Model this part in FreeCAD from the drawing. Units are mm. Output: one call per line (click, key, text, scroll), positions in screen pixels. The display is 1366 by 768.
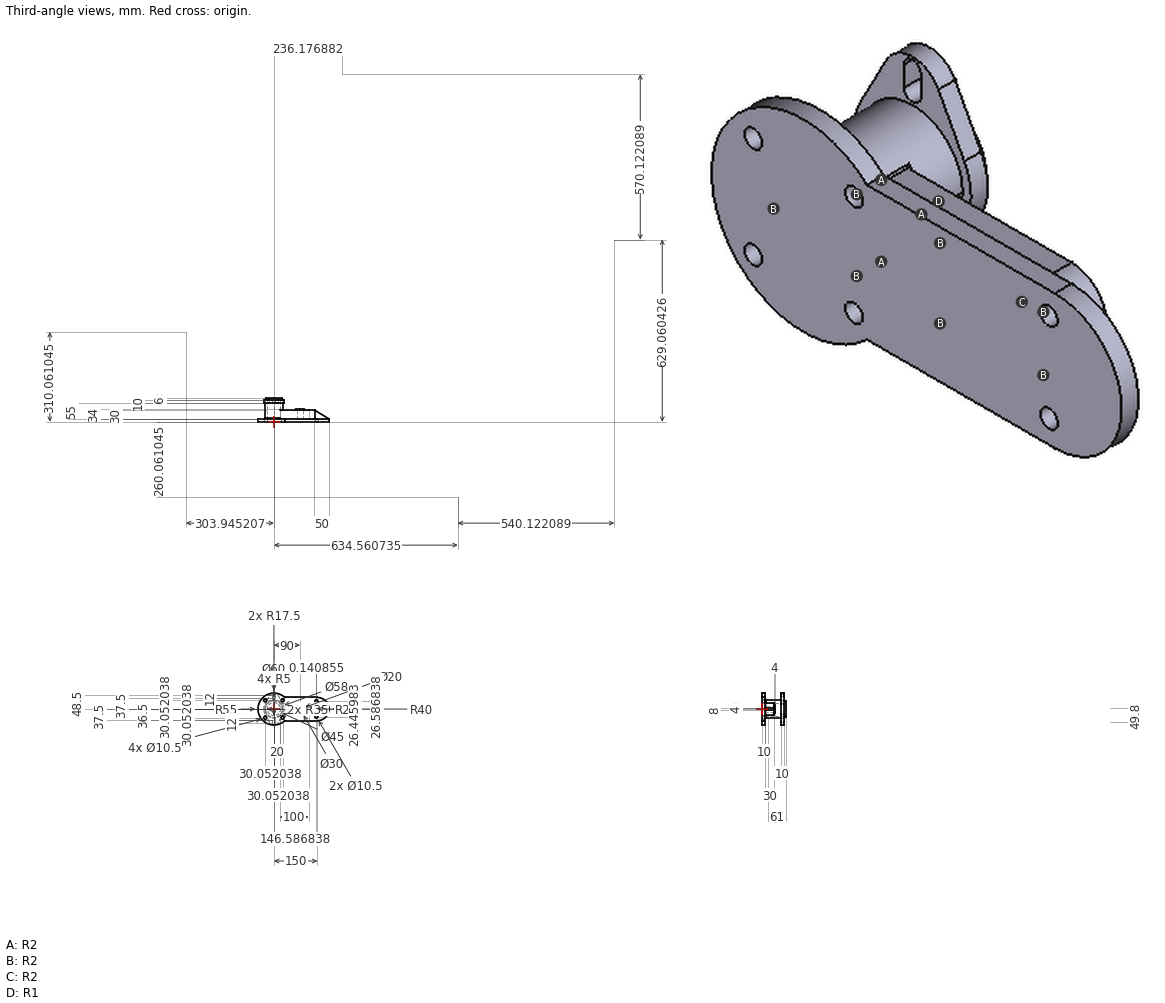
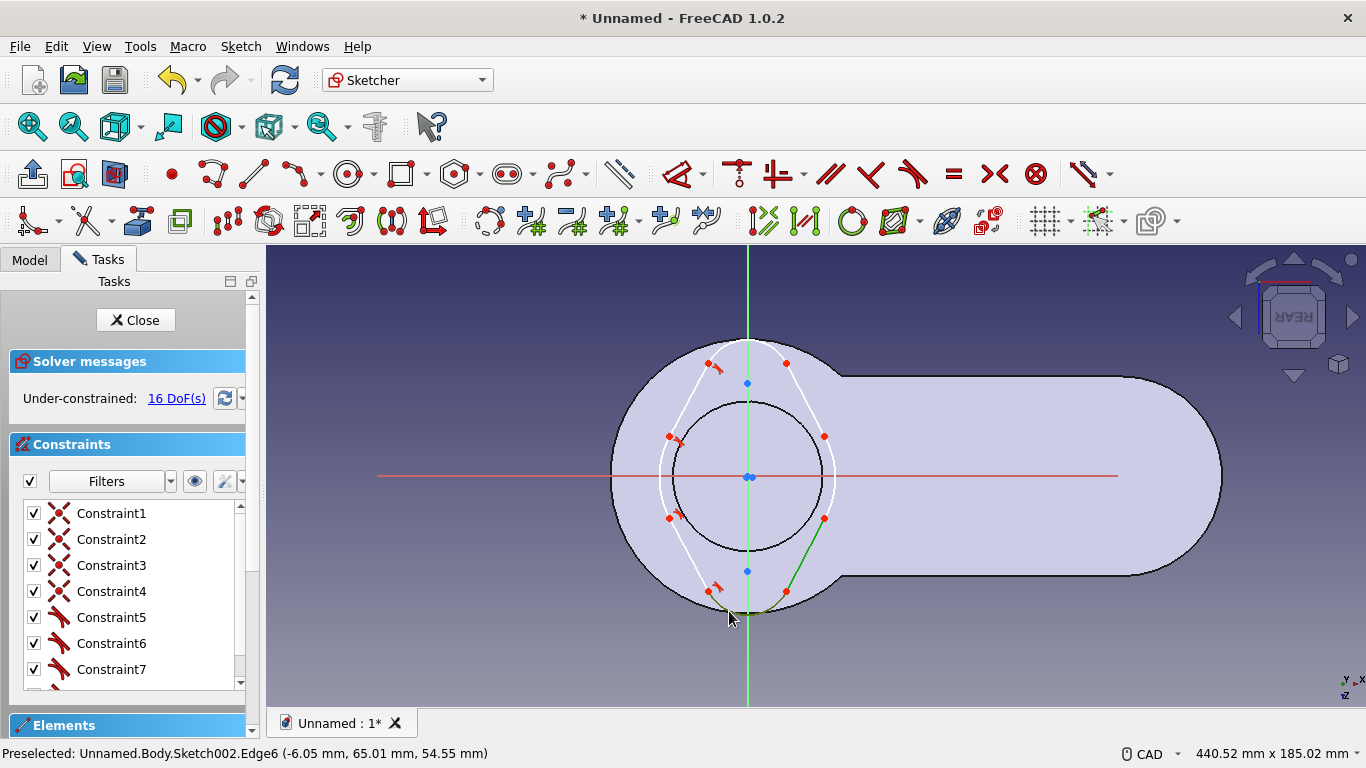
key(t)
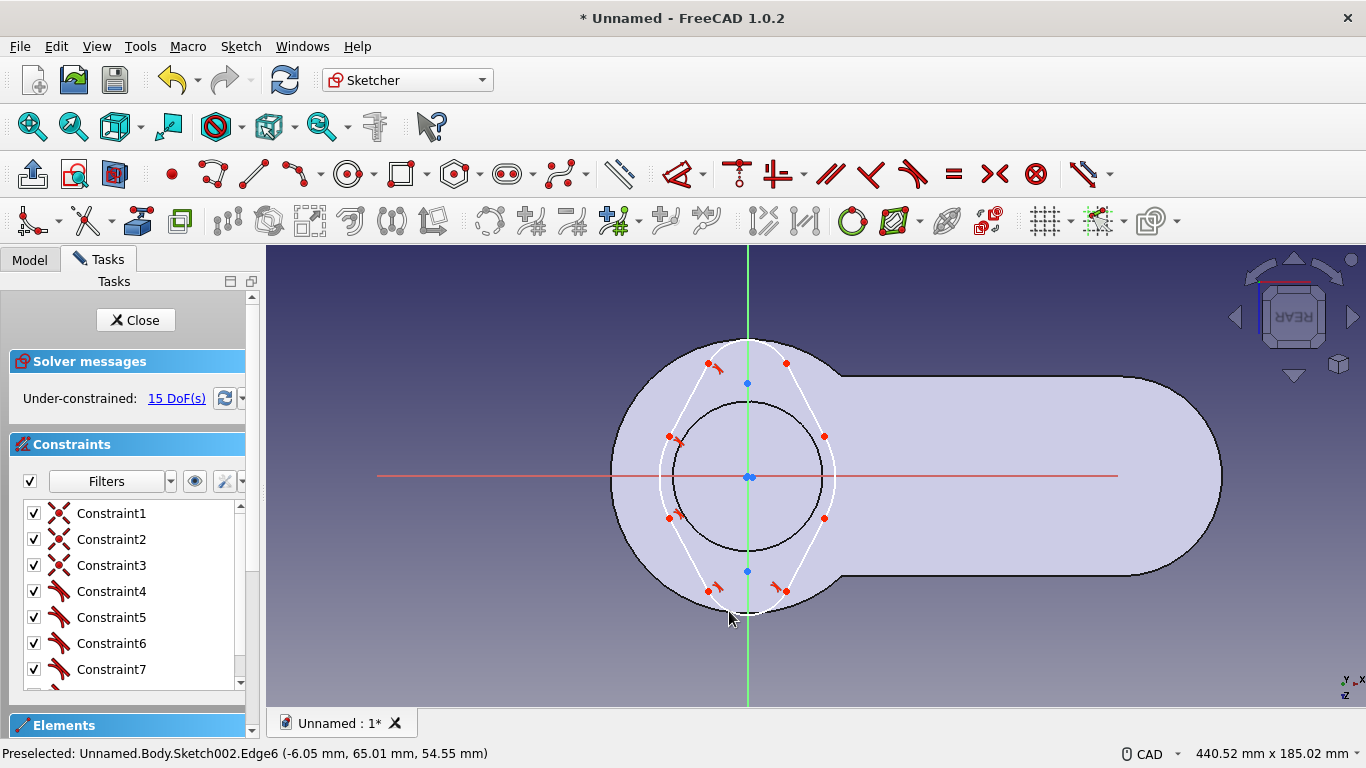
click(798, 570)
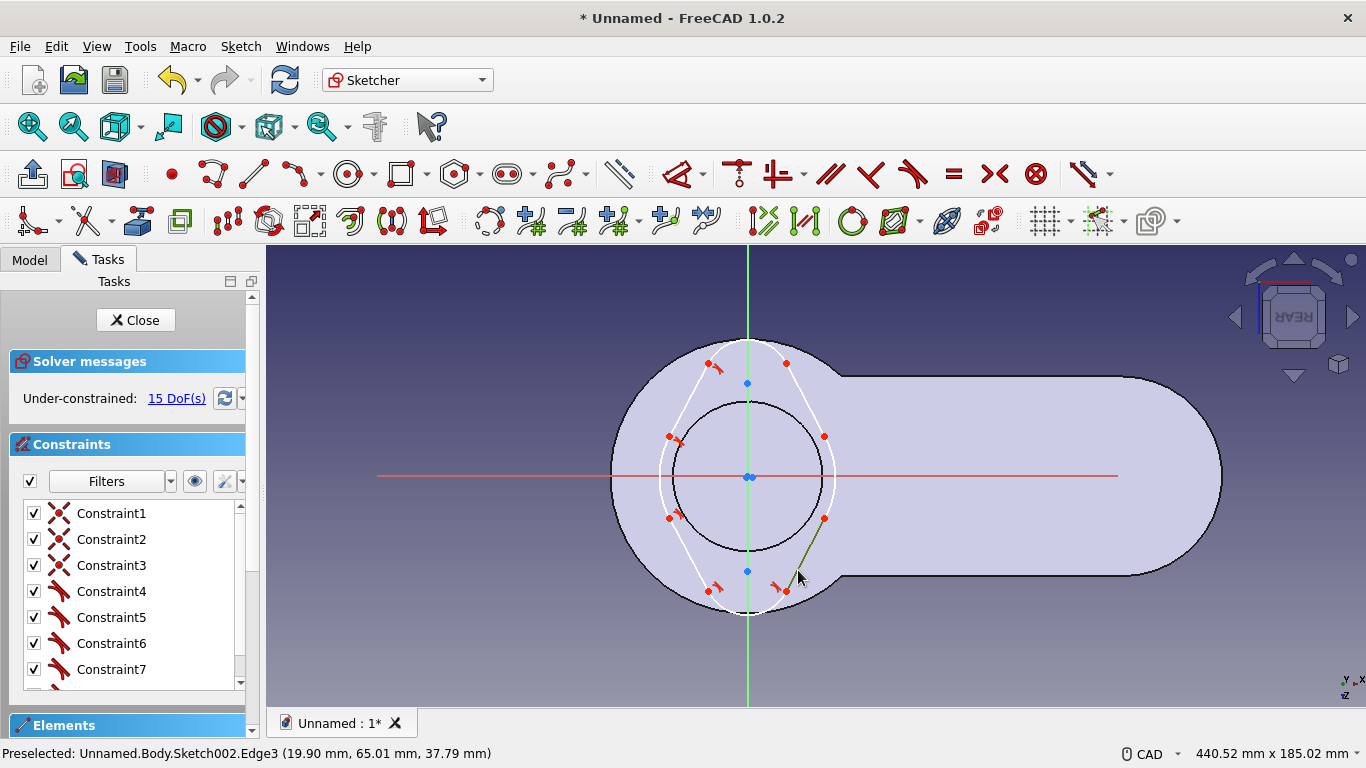
click(834, 495)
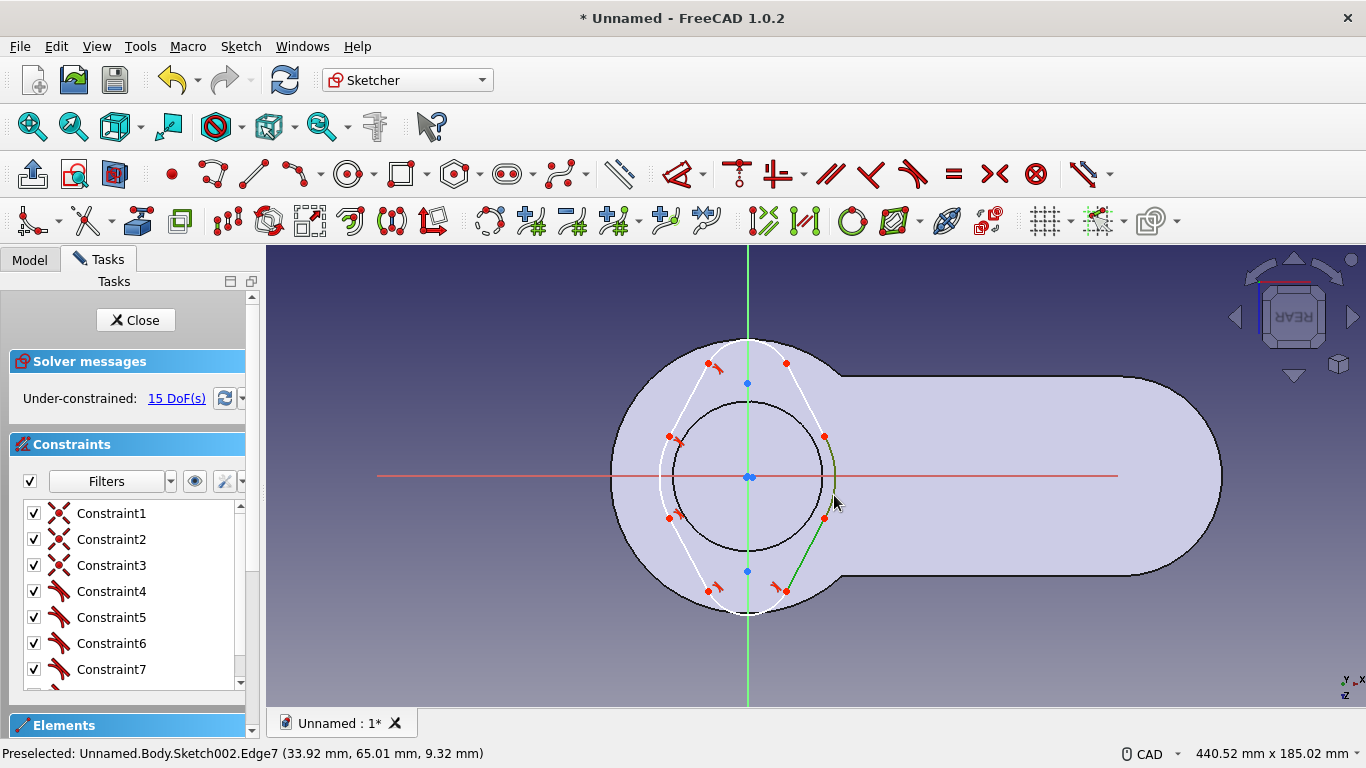
key(t)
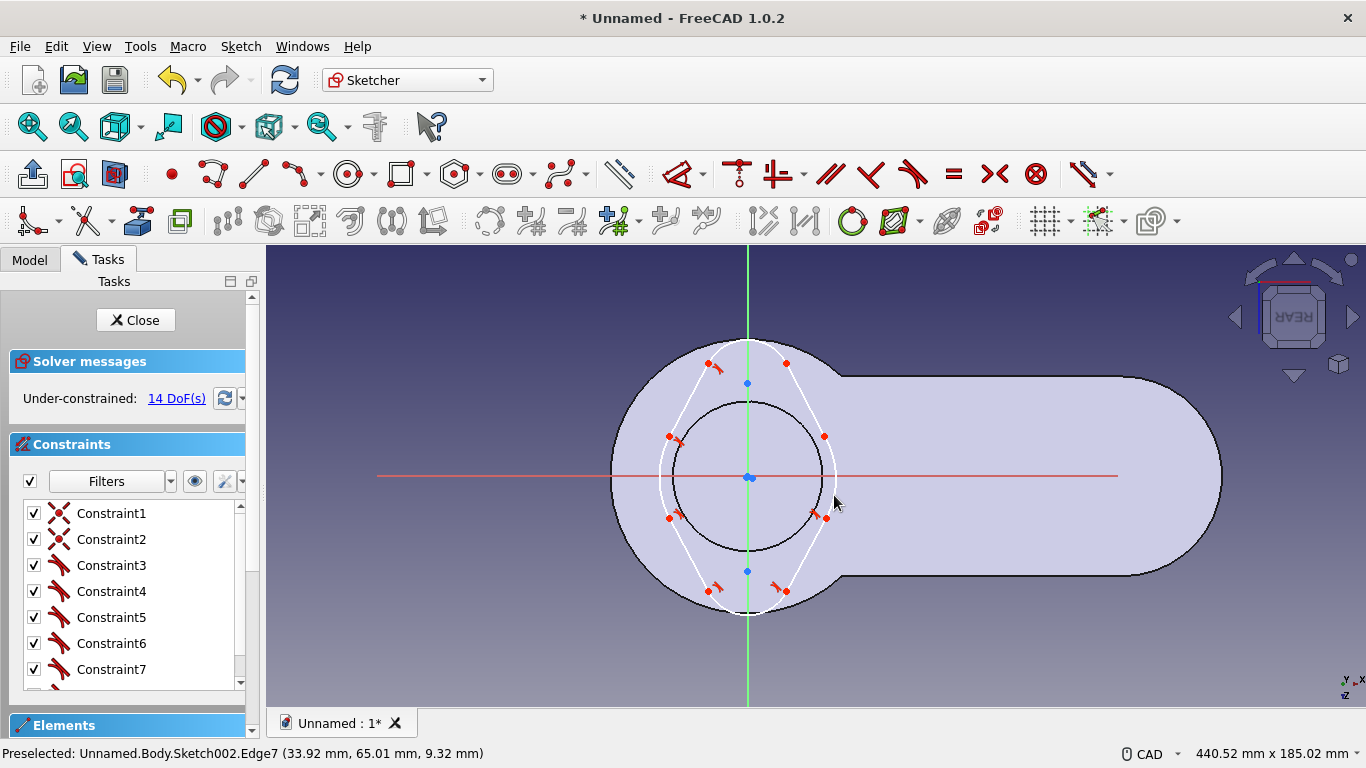
click(813, 415)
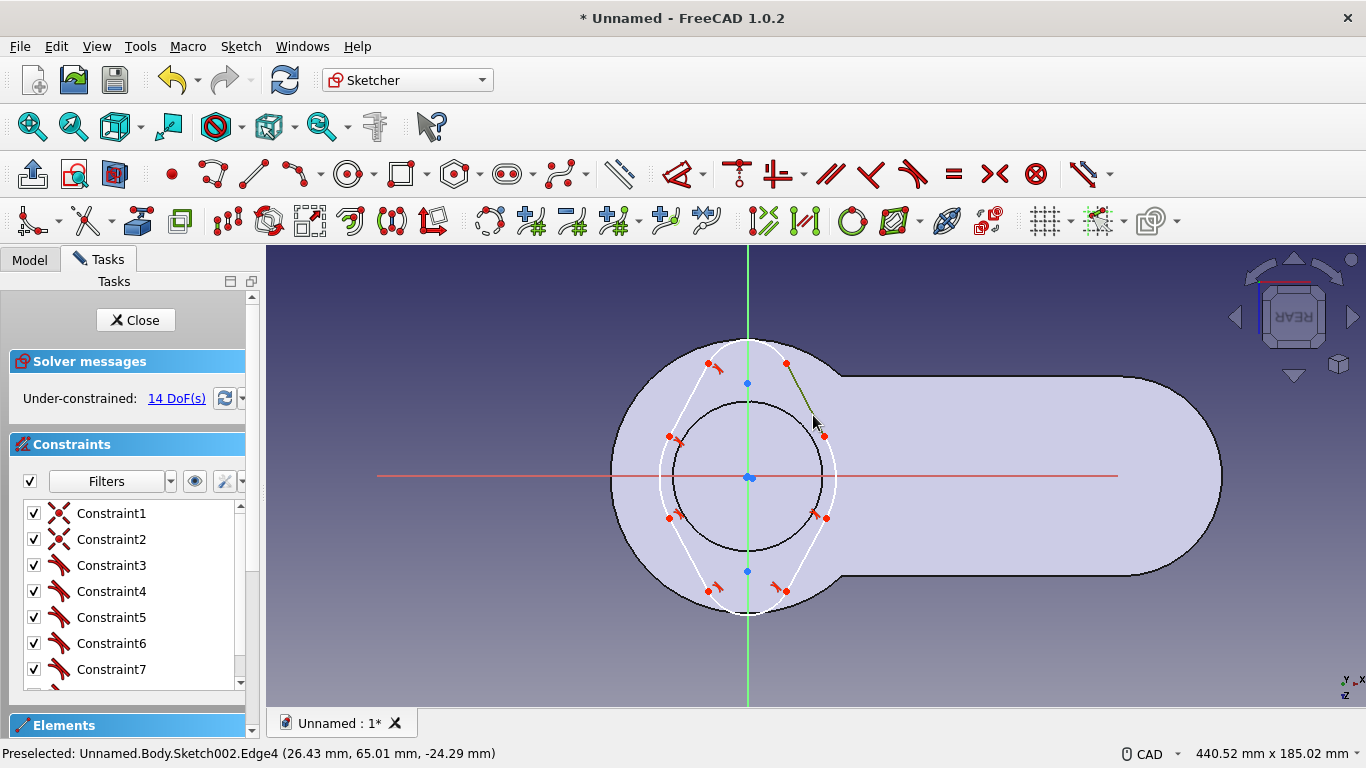
click(835, 494)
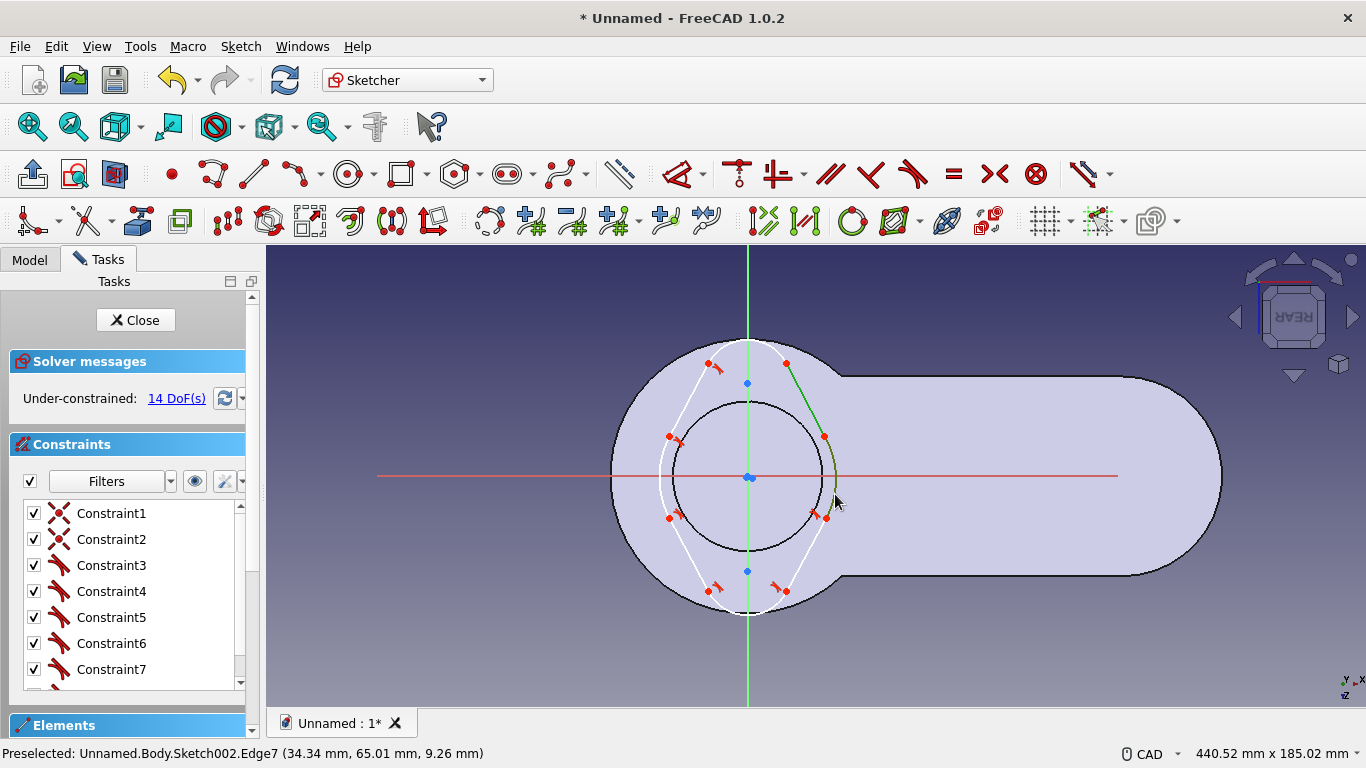
key(t)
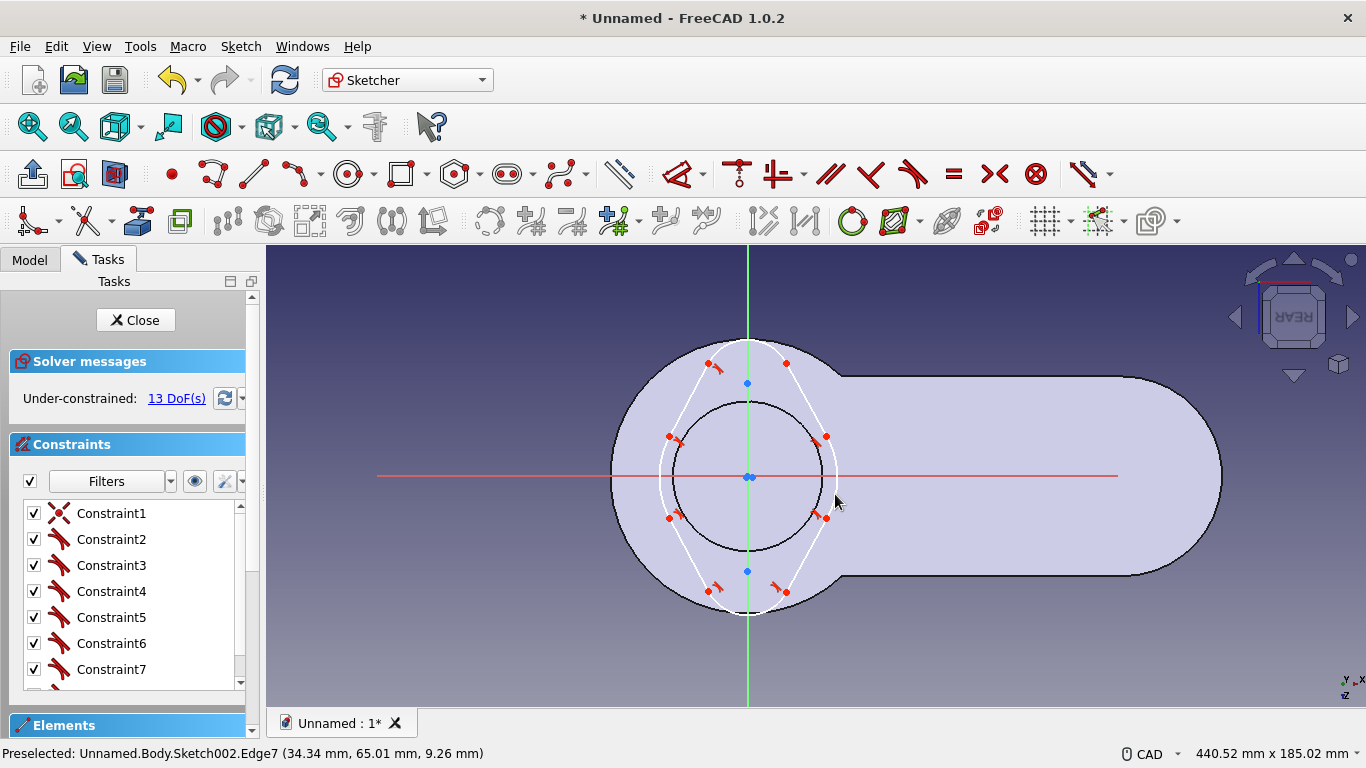
click(815, 415)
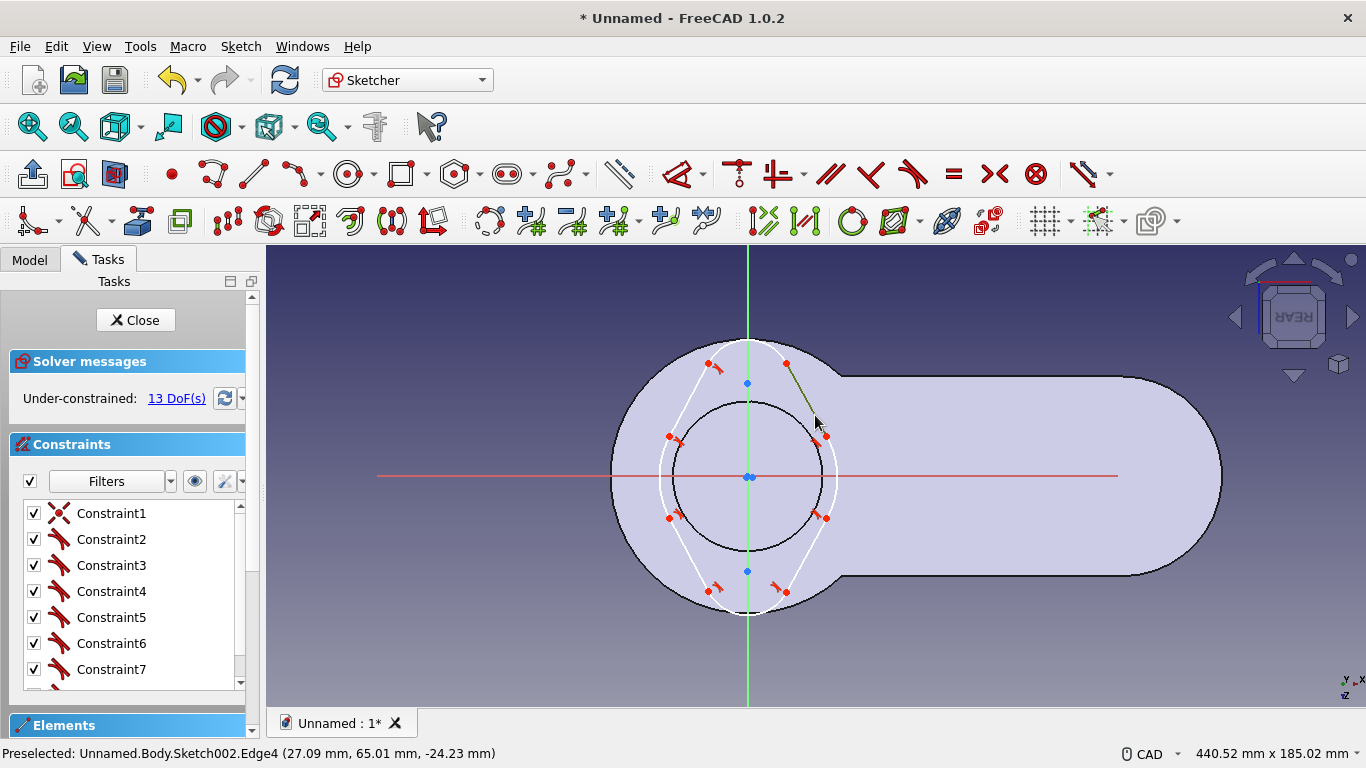
click(766, 344)